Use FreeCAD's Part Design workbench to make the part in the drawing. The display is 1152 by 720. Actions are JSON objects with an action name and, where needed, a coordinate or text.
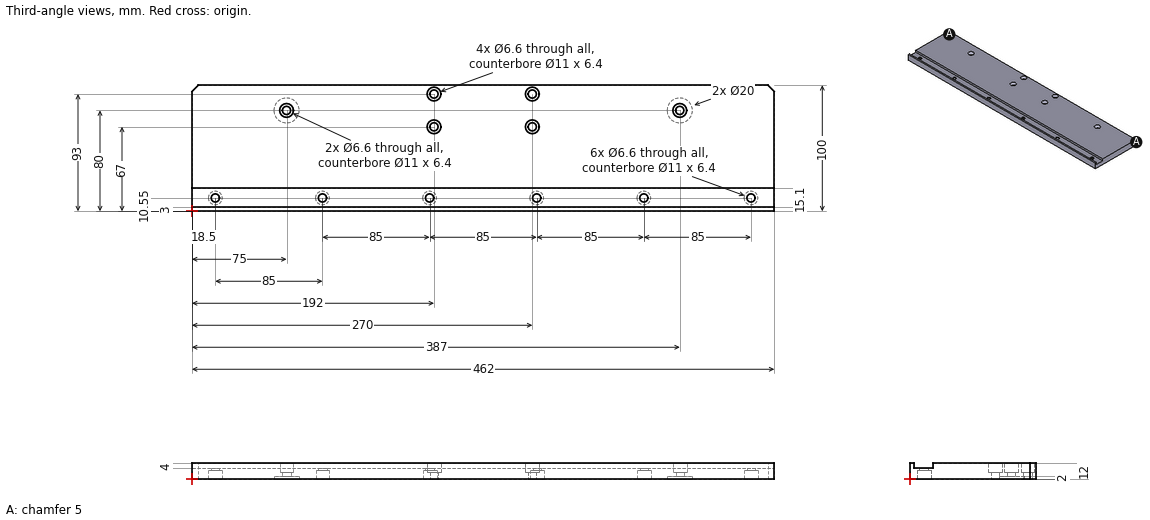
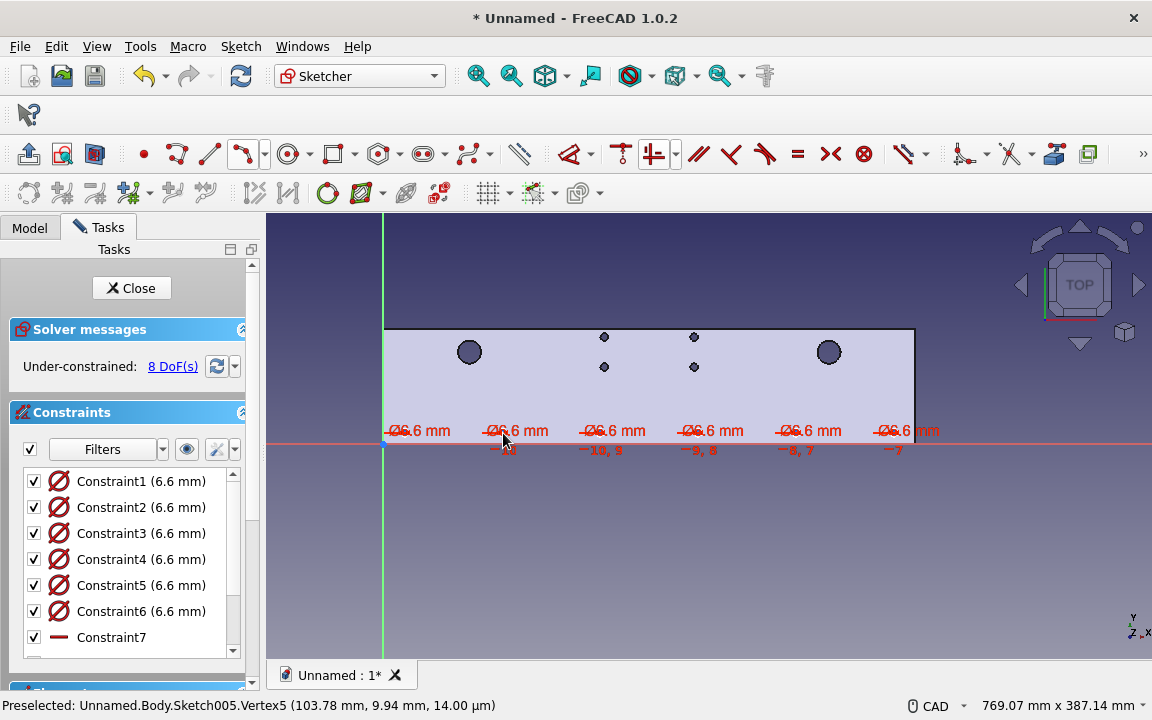
{"action": "left_click", "coordinate": [503, 433]}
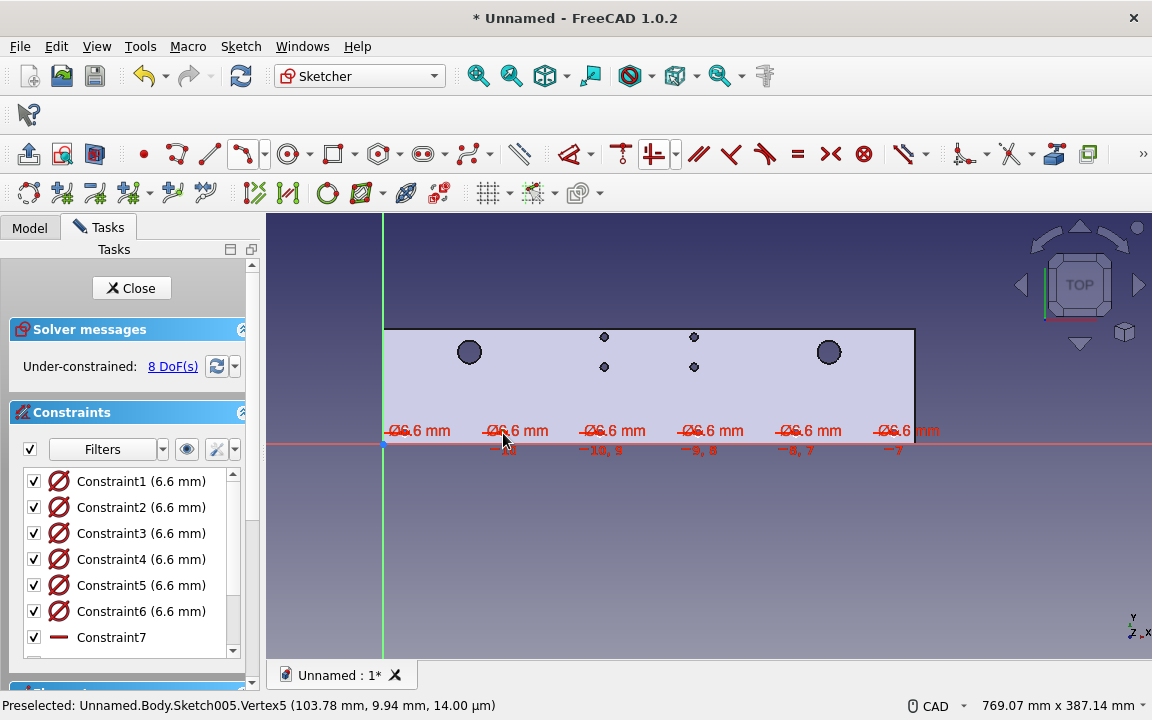
{"action": "left_click", "coordinate": [405, 433]}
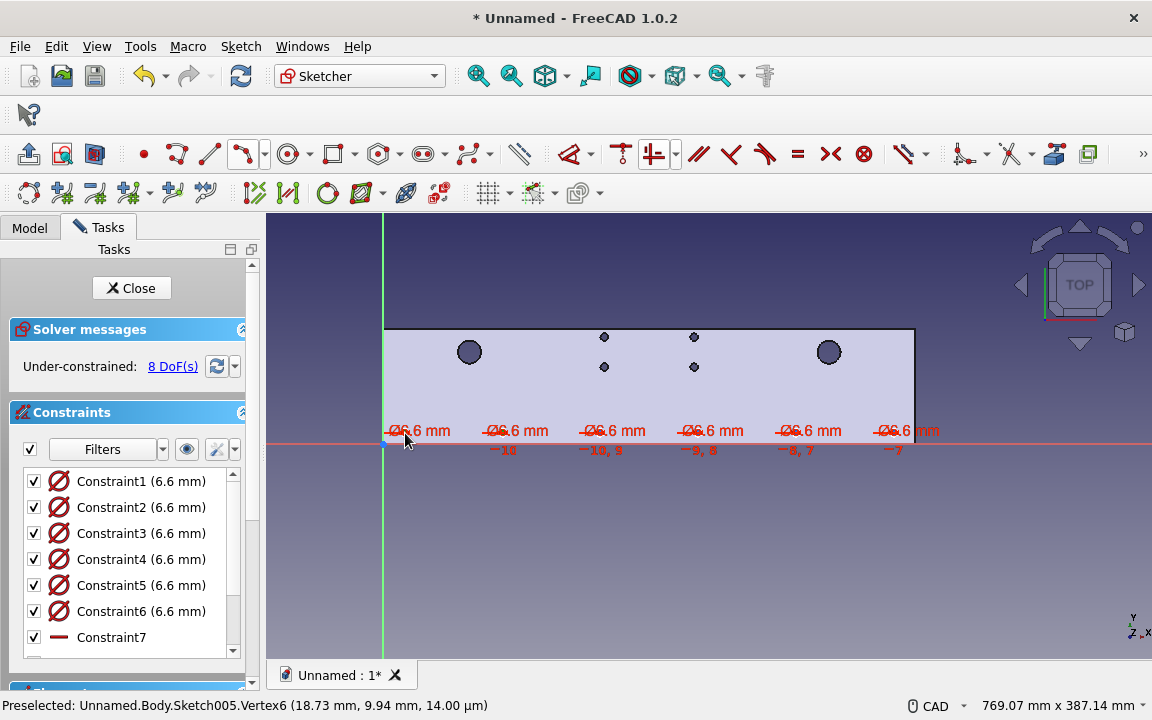
{"action": "left_click", "coordinate": [676, 154]}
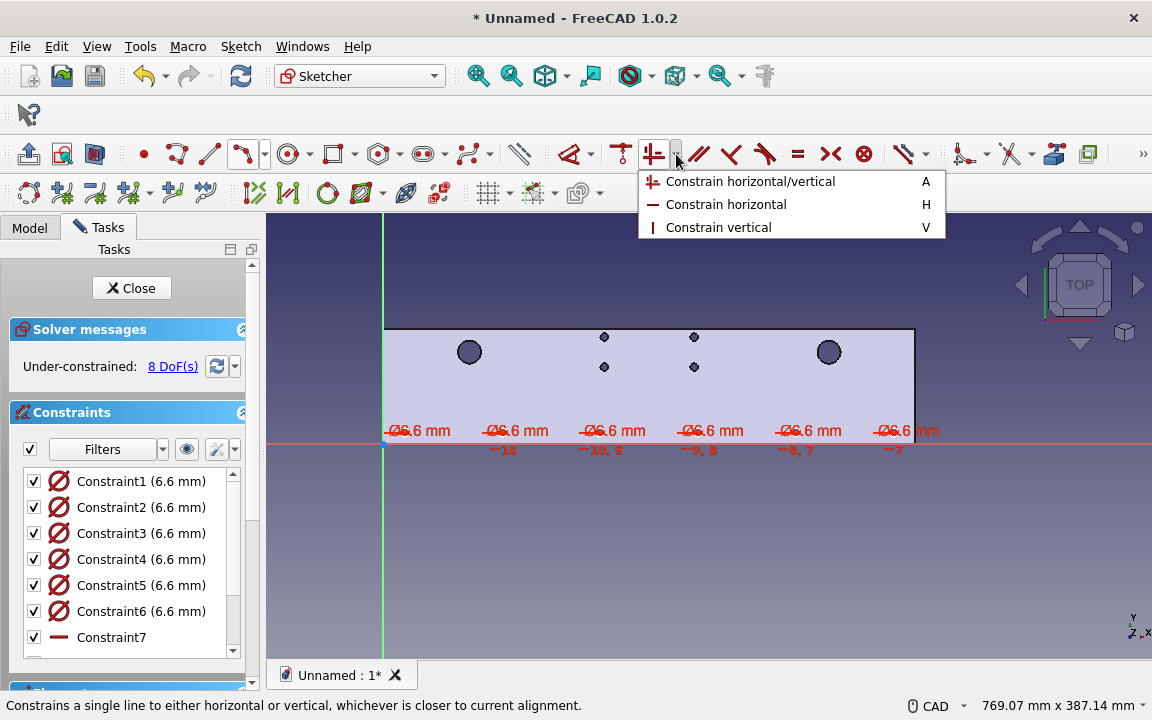
{"action": "left_click", "coordinate": [792, 204]}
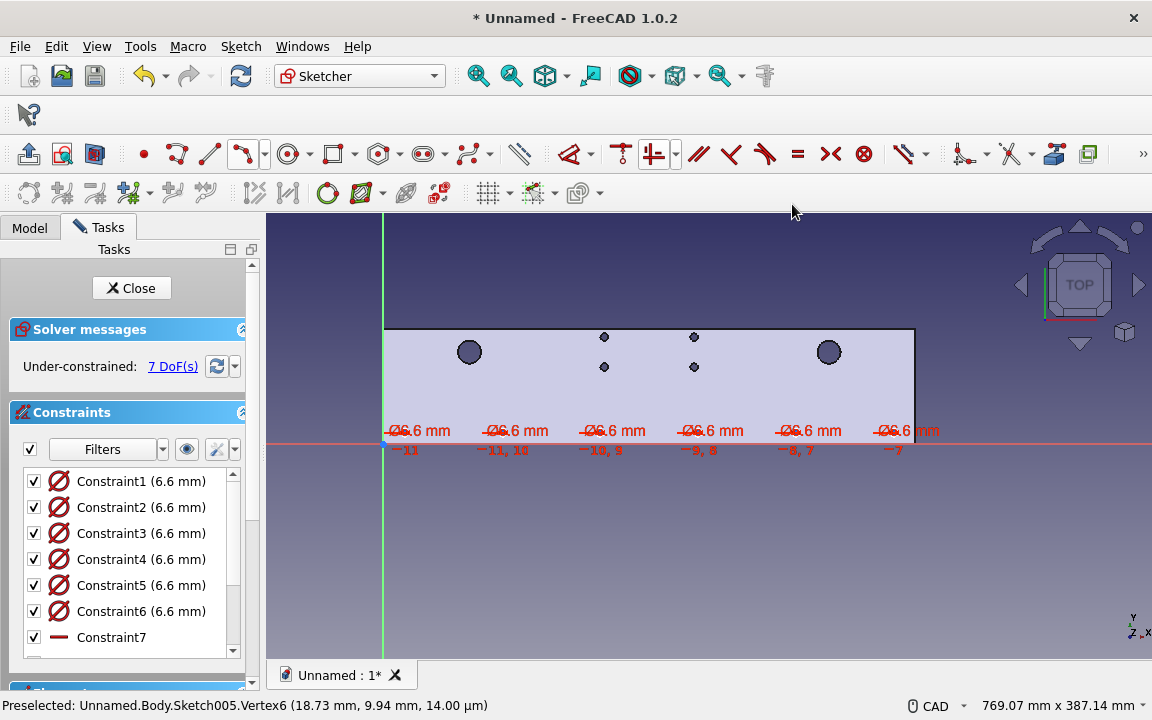
{"action": "left_click", "coordinate": [568, 154]}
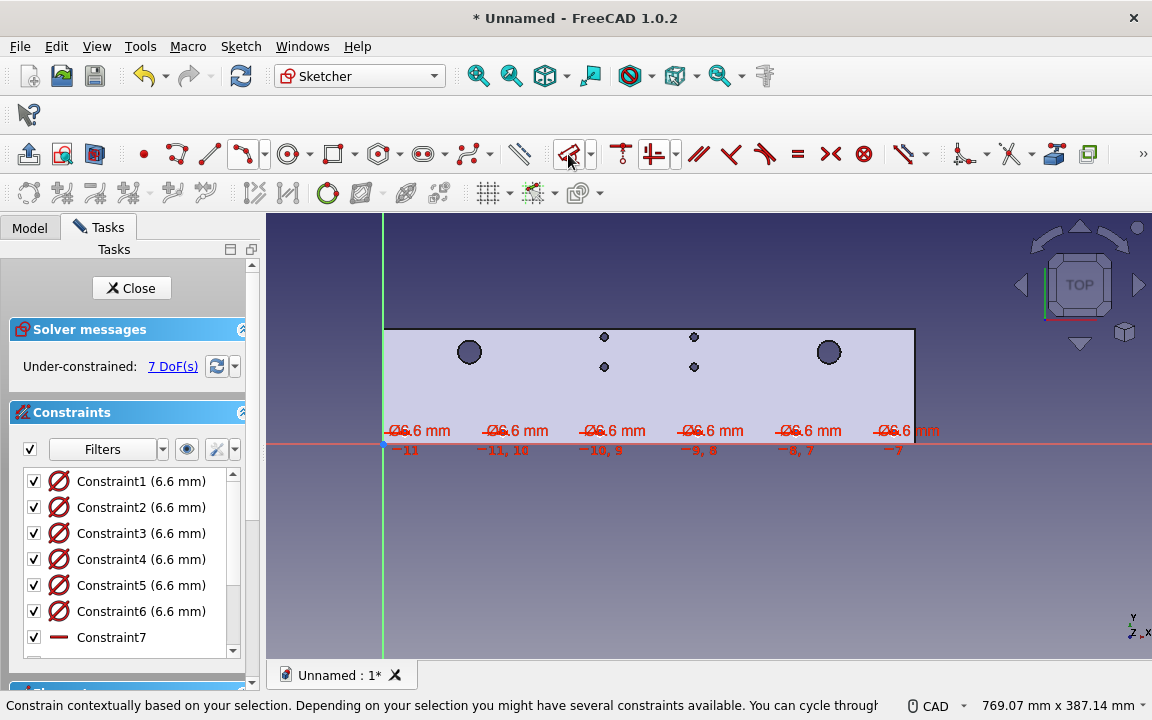
{"action": "left_click", "coordinate": [894, 433]}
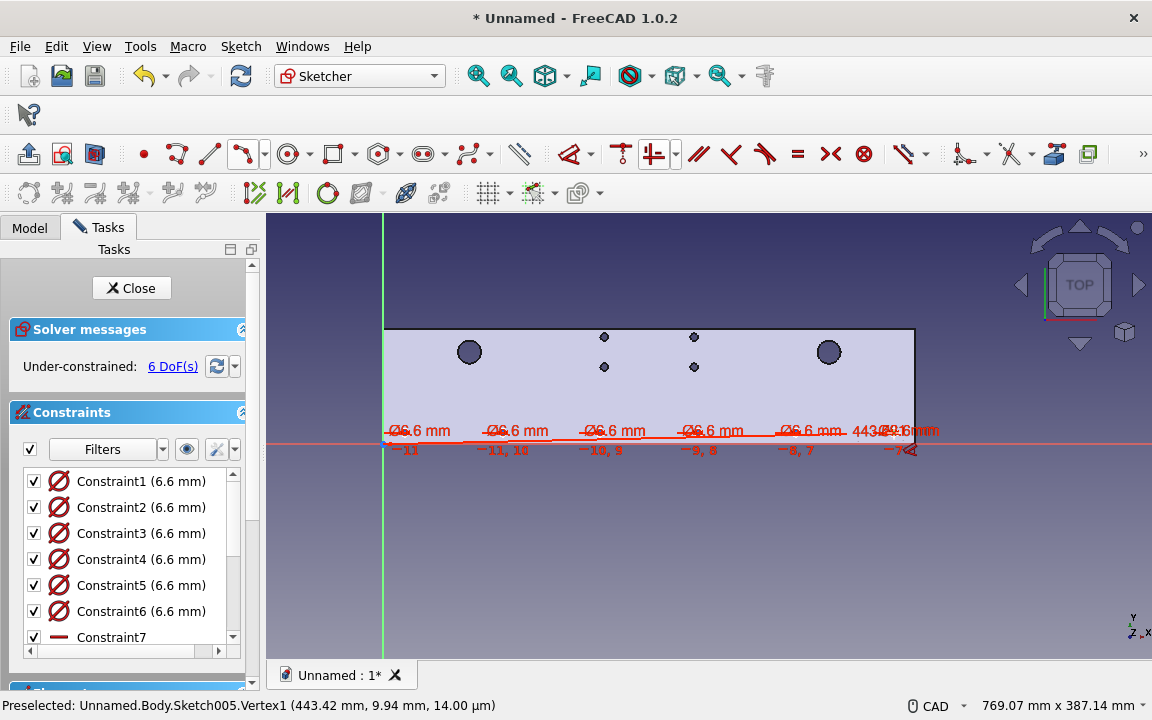
{"action": "left_click", "coordinate": [796, 433]}
{"action": "left_click", "coordinate": [845, 399]}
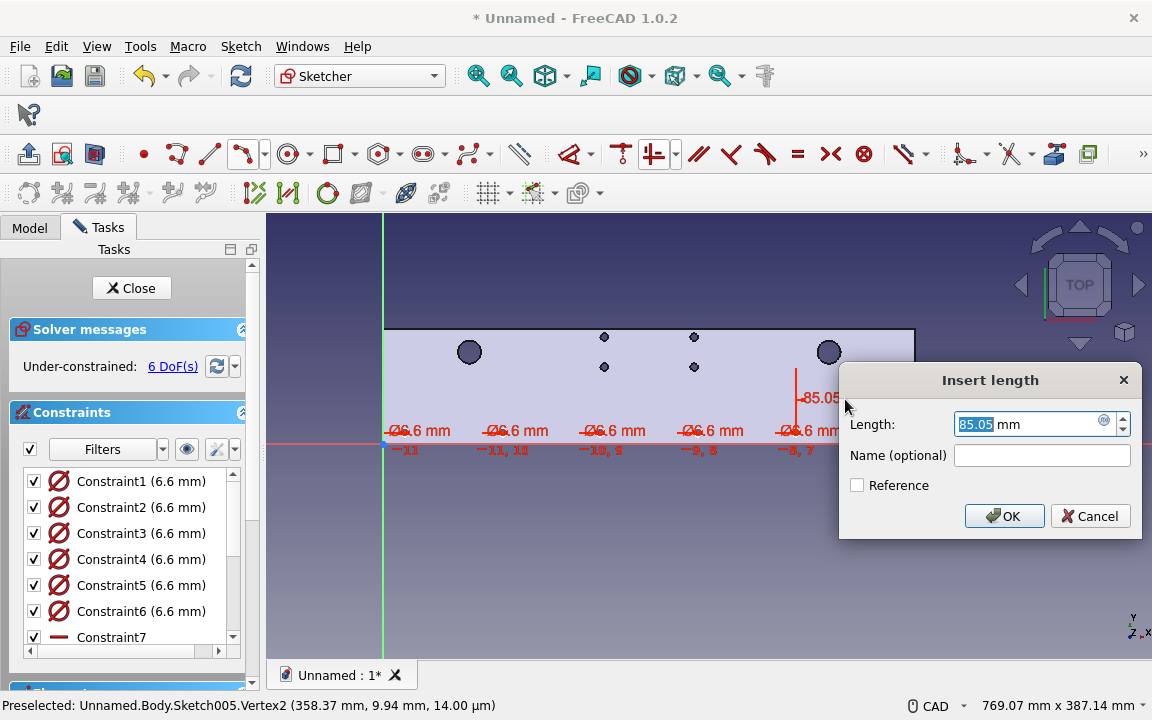
{"action": "type", "text": "85"}
{"action": "key", "text": "Return"}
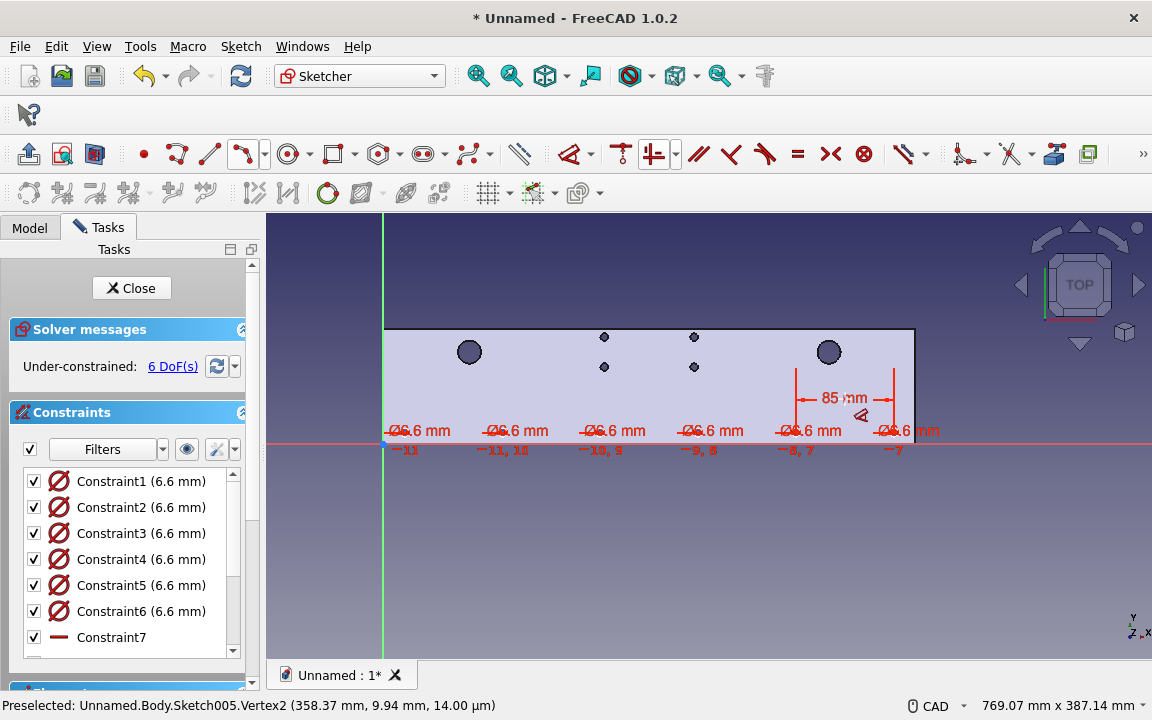
{"action": "left_click", "coordinate": [796, 433]}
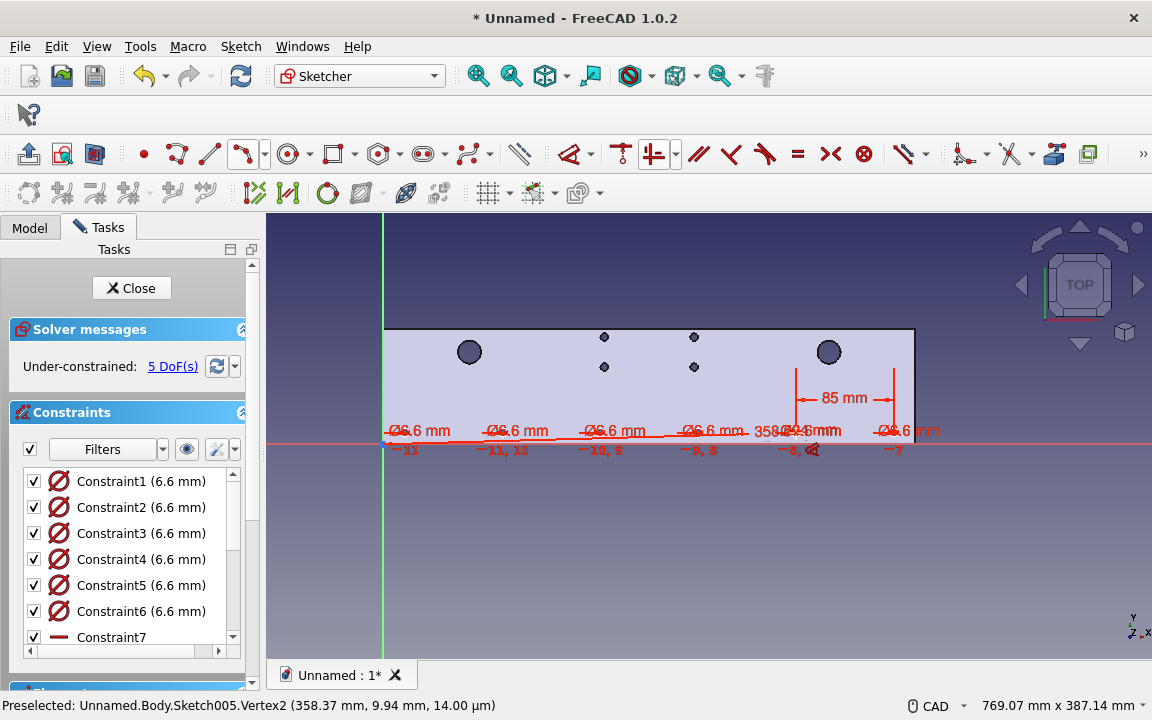
{"action": "left_click", "coordinate": [698, 433]}
{"action": "left_click", "coordinate": [747, 399]}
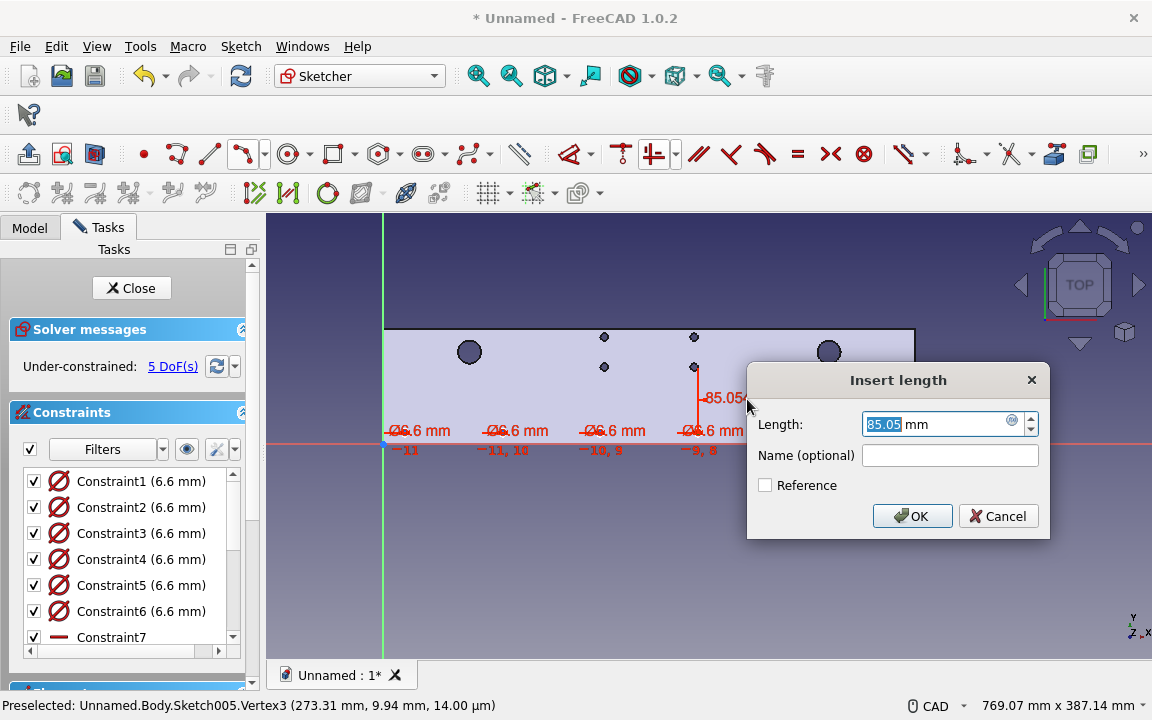
{"action": "type", "text": "85"}
{"action": "key", "text": "Return"}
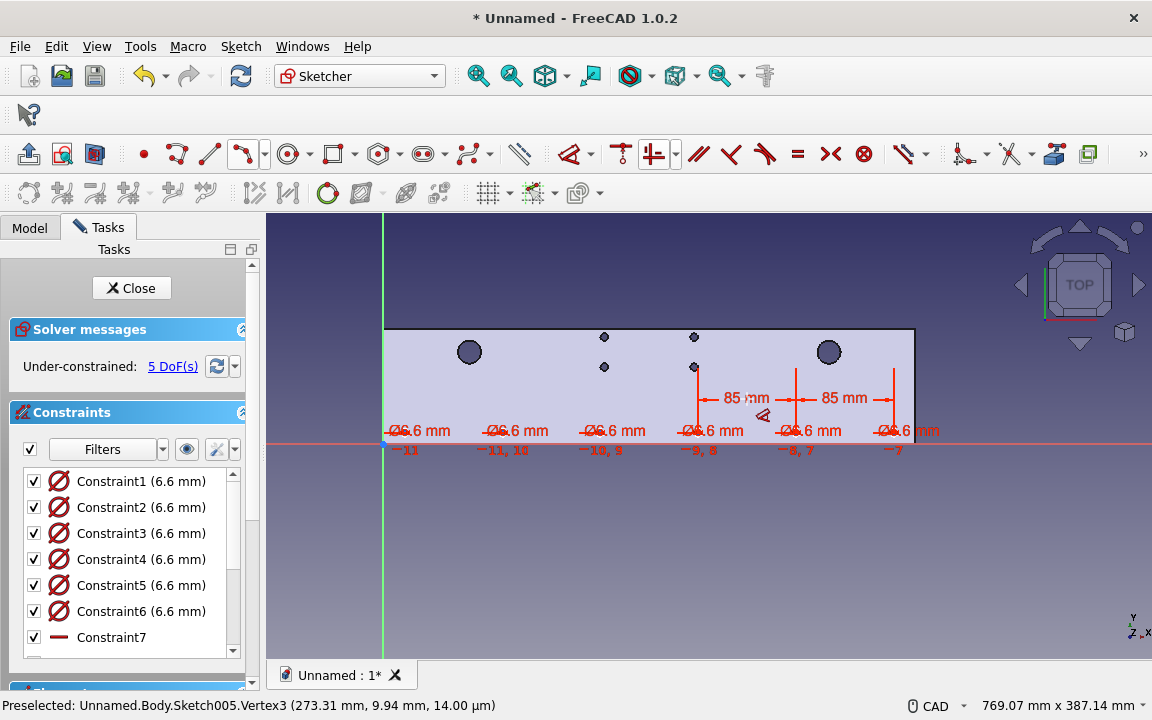
{"action": "left_click", "coordinate": [698, 433]}